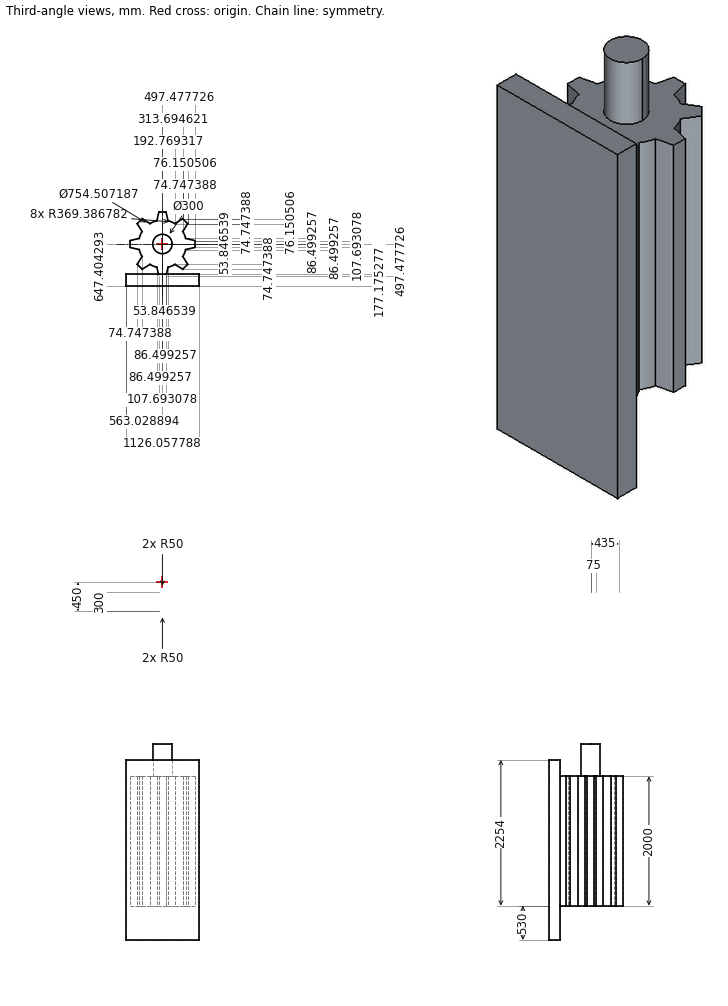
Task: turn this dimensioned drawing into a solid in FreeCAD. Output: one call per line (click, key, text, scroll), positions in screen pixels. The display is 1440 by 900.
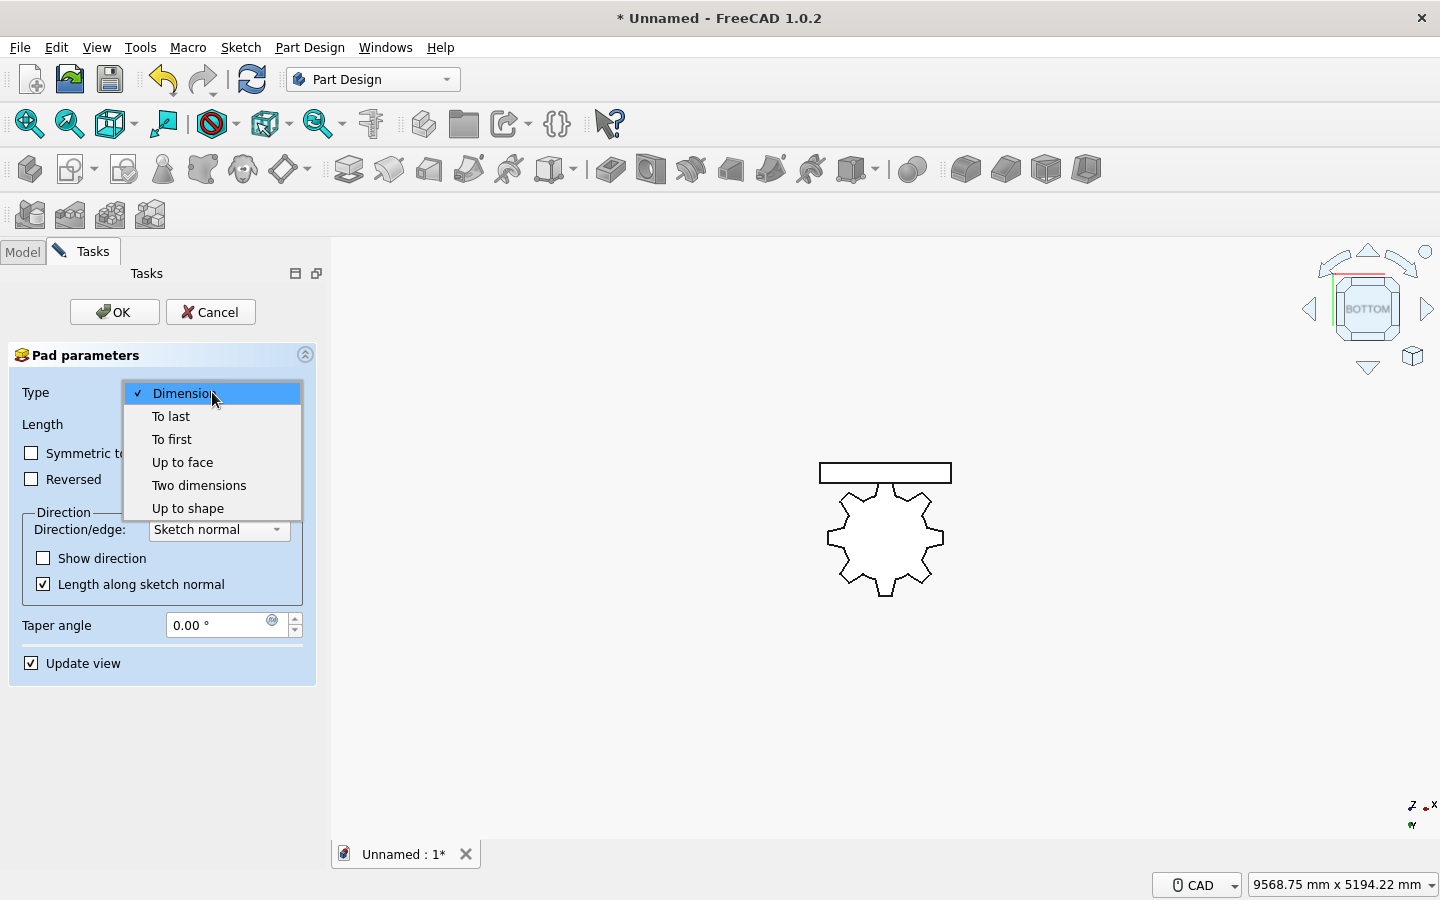
click(212, 486)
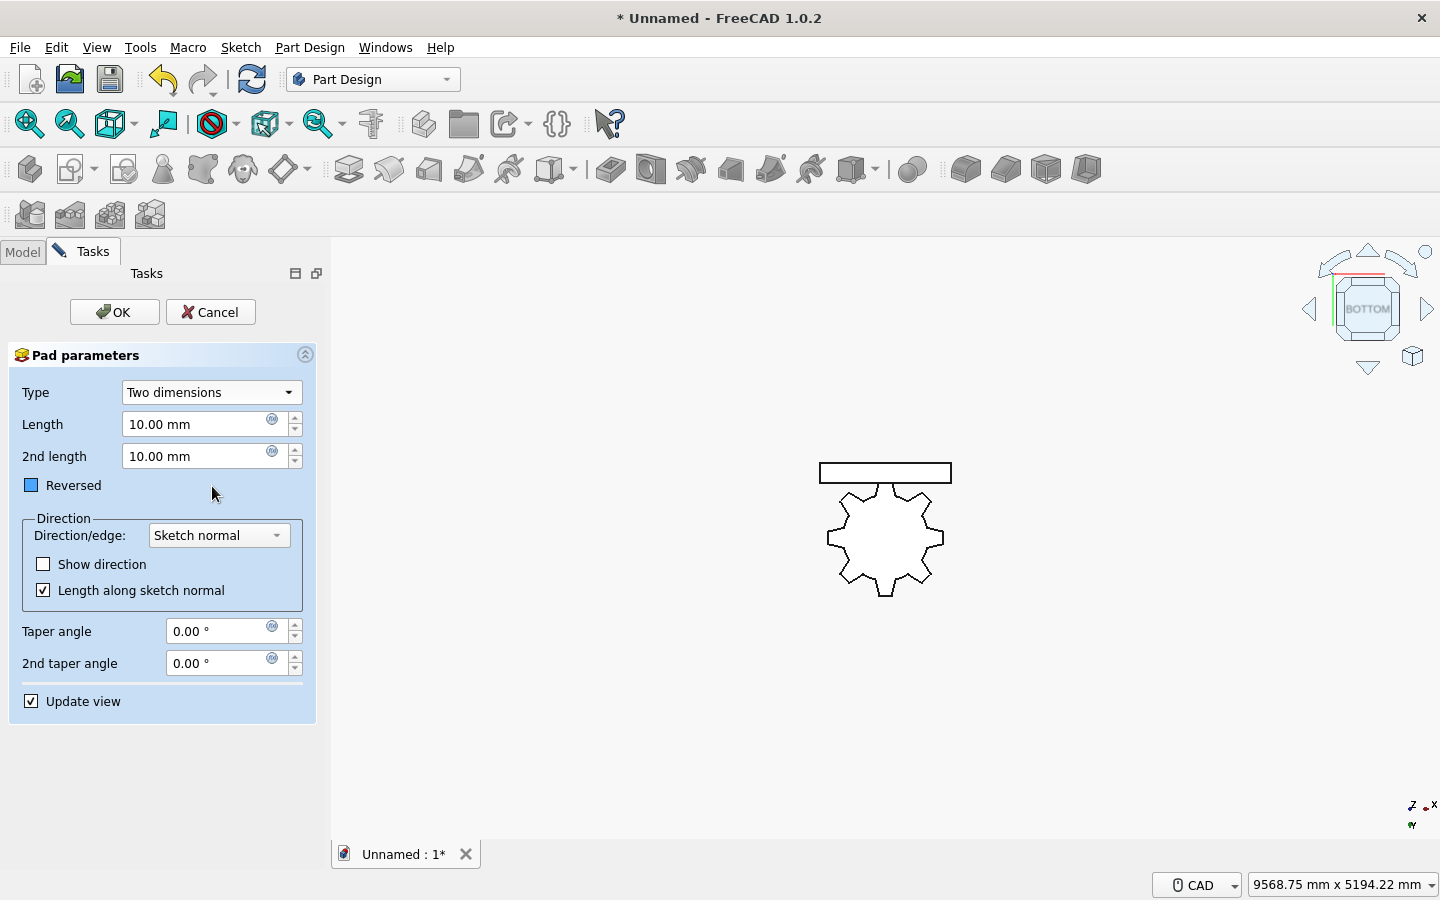
triple_click(204, 424)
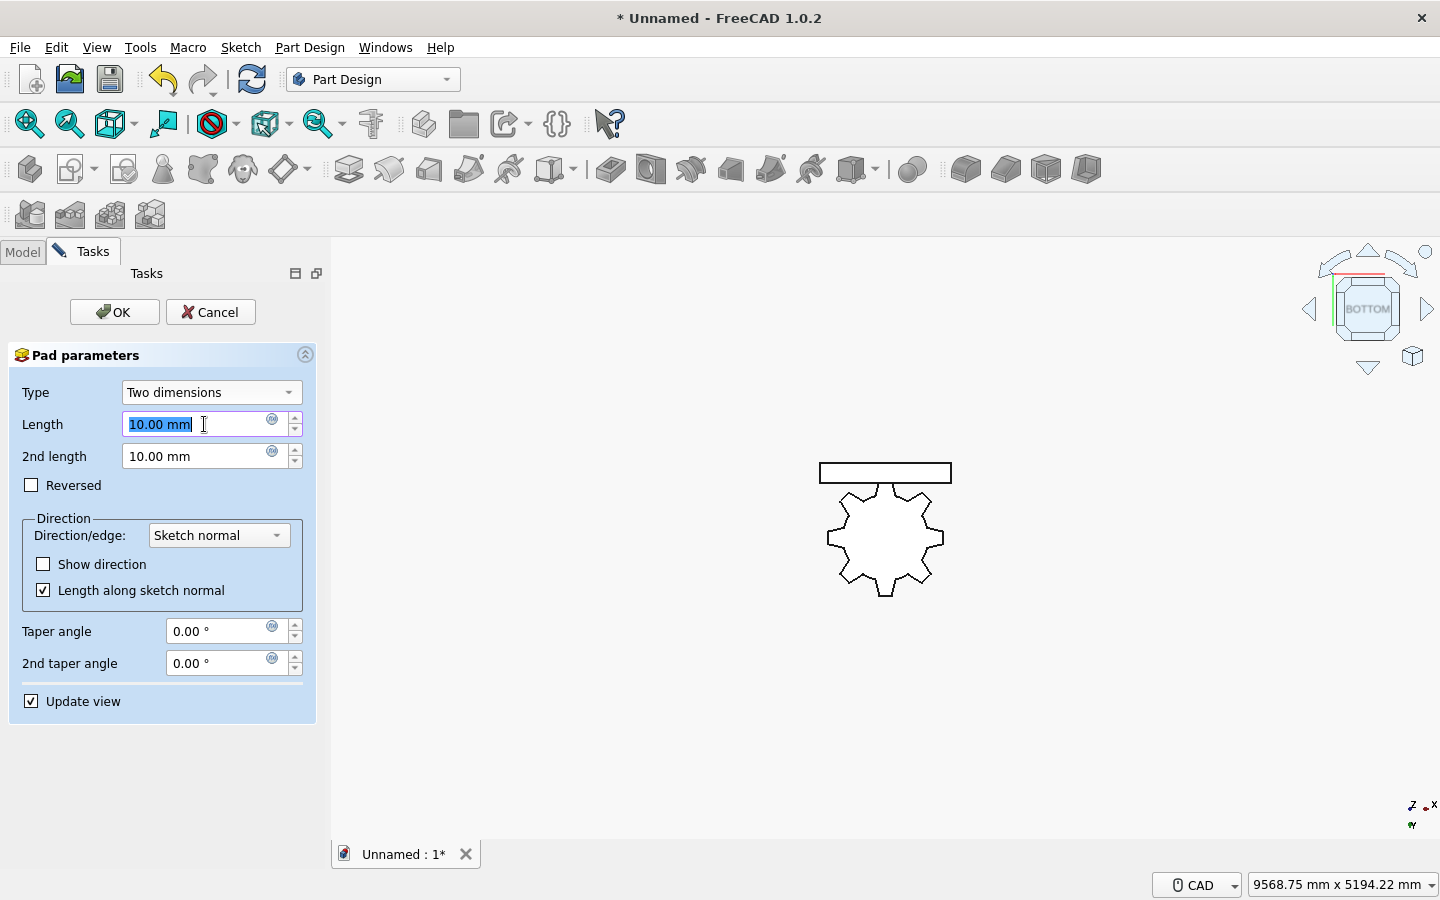
text(530)
key(Tab)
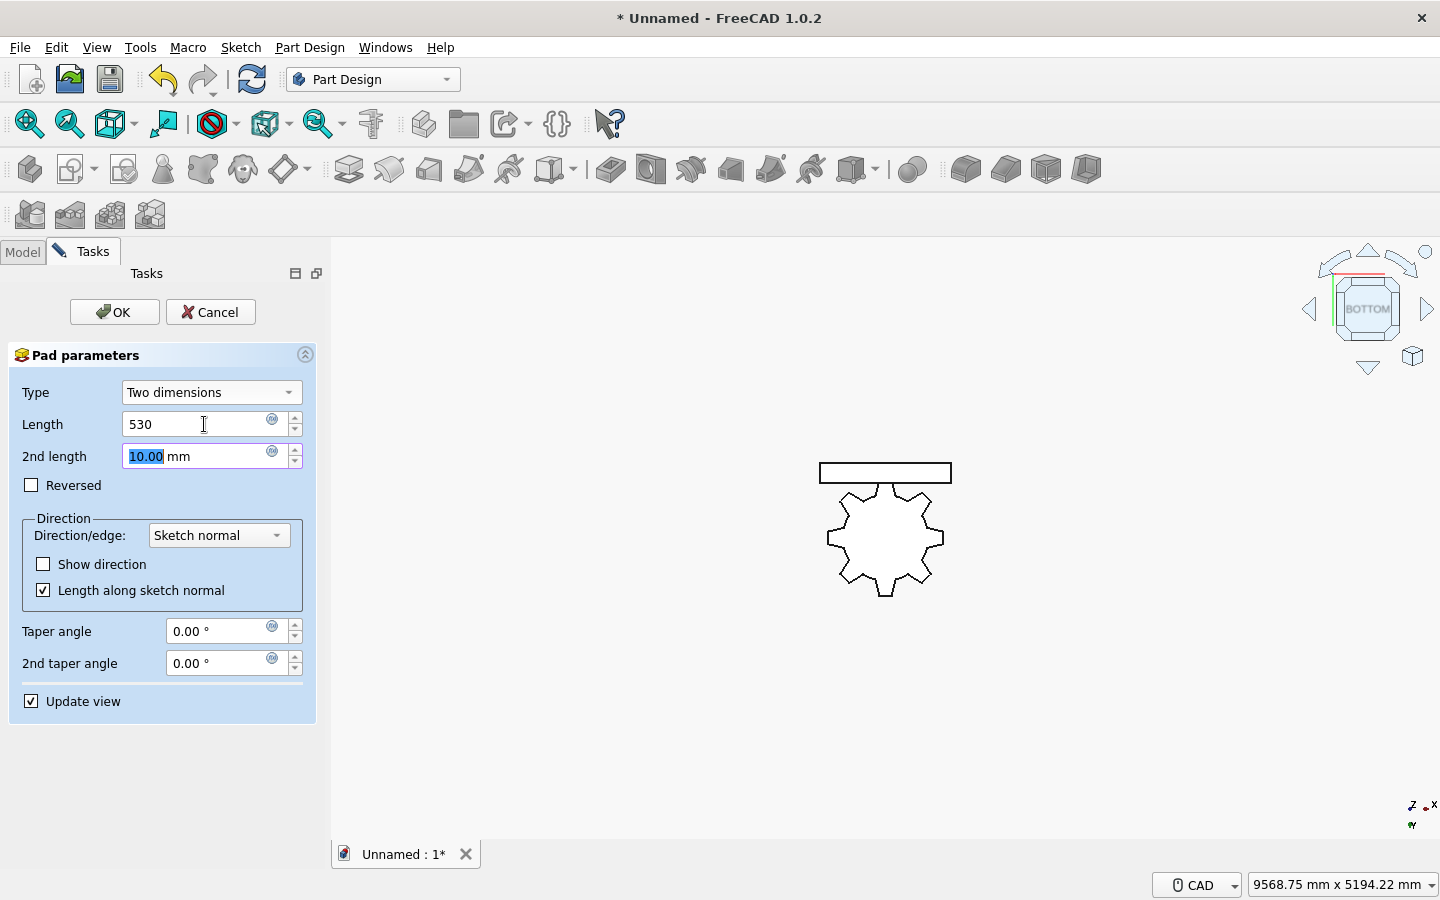
text(2254)
key(Tab)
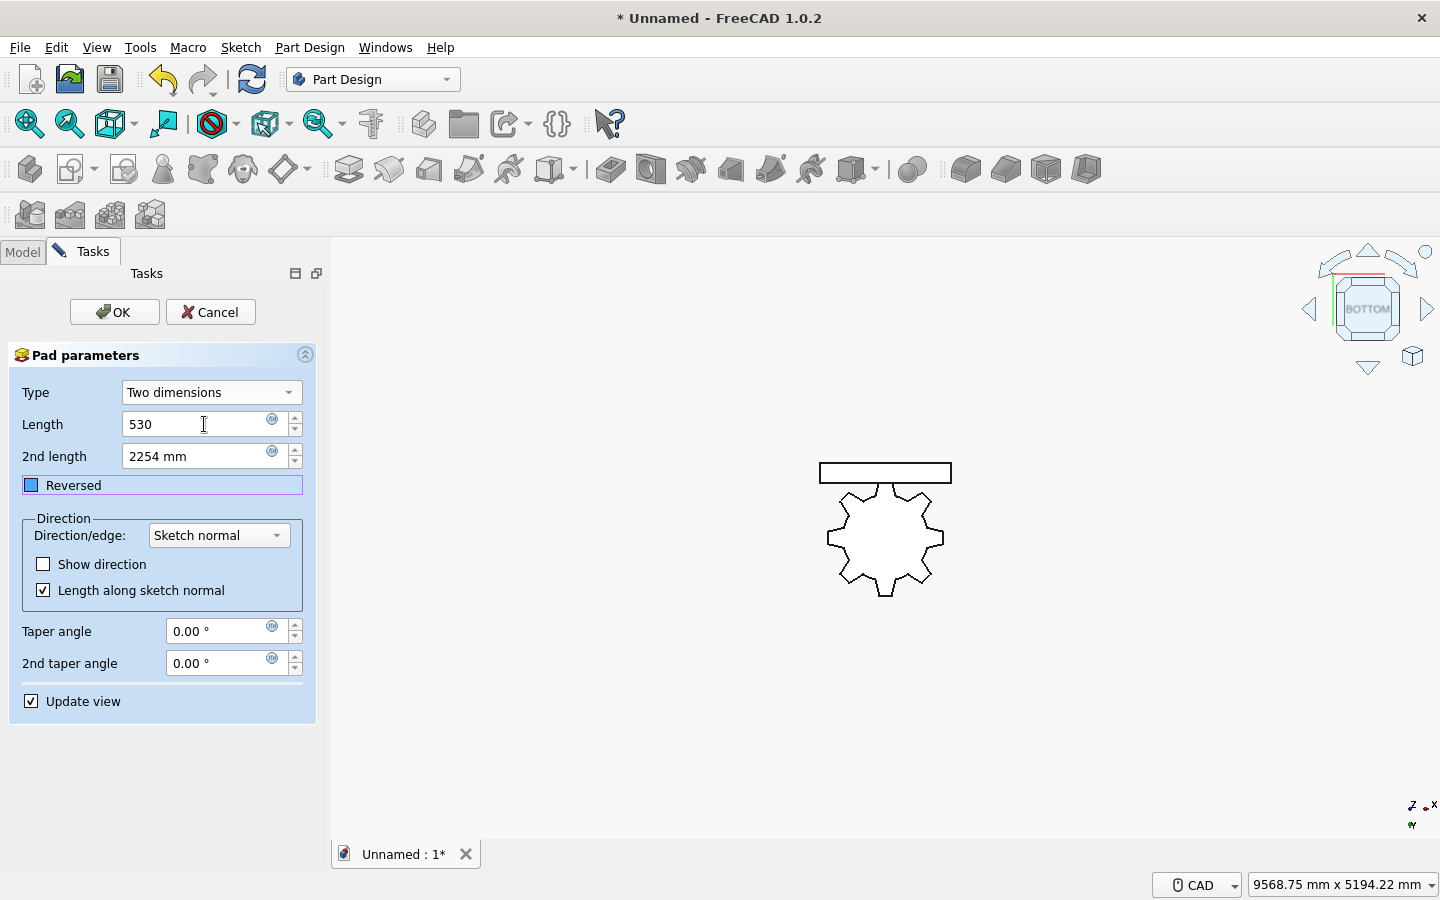
click(115, 312)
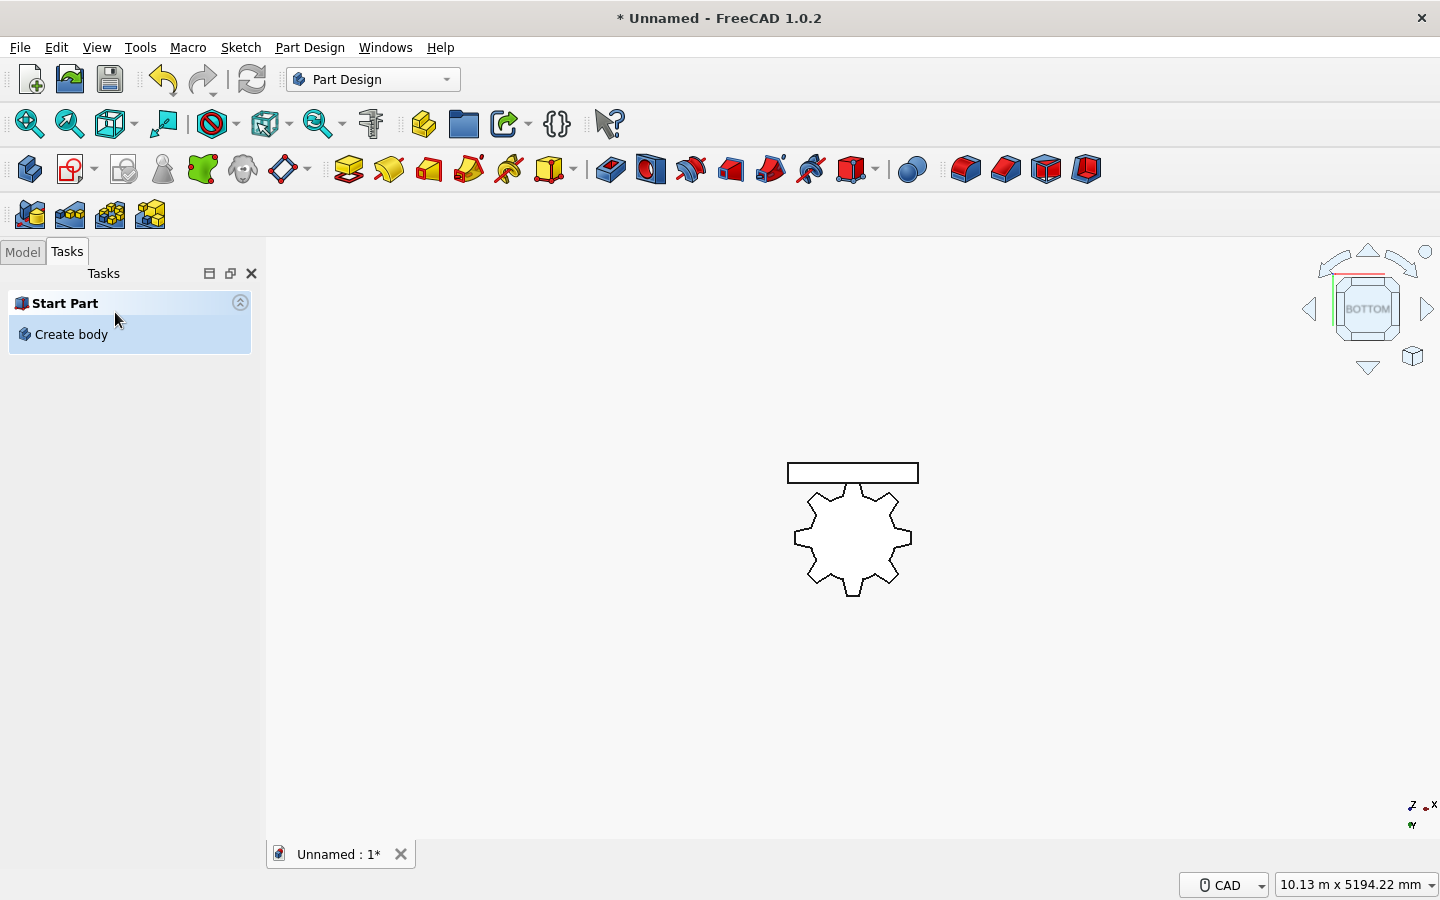
click(30, 124)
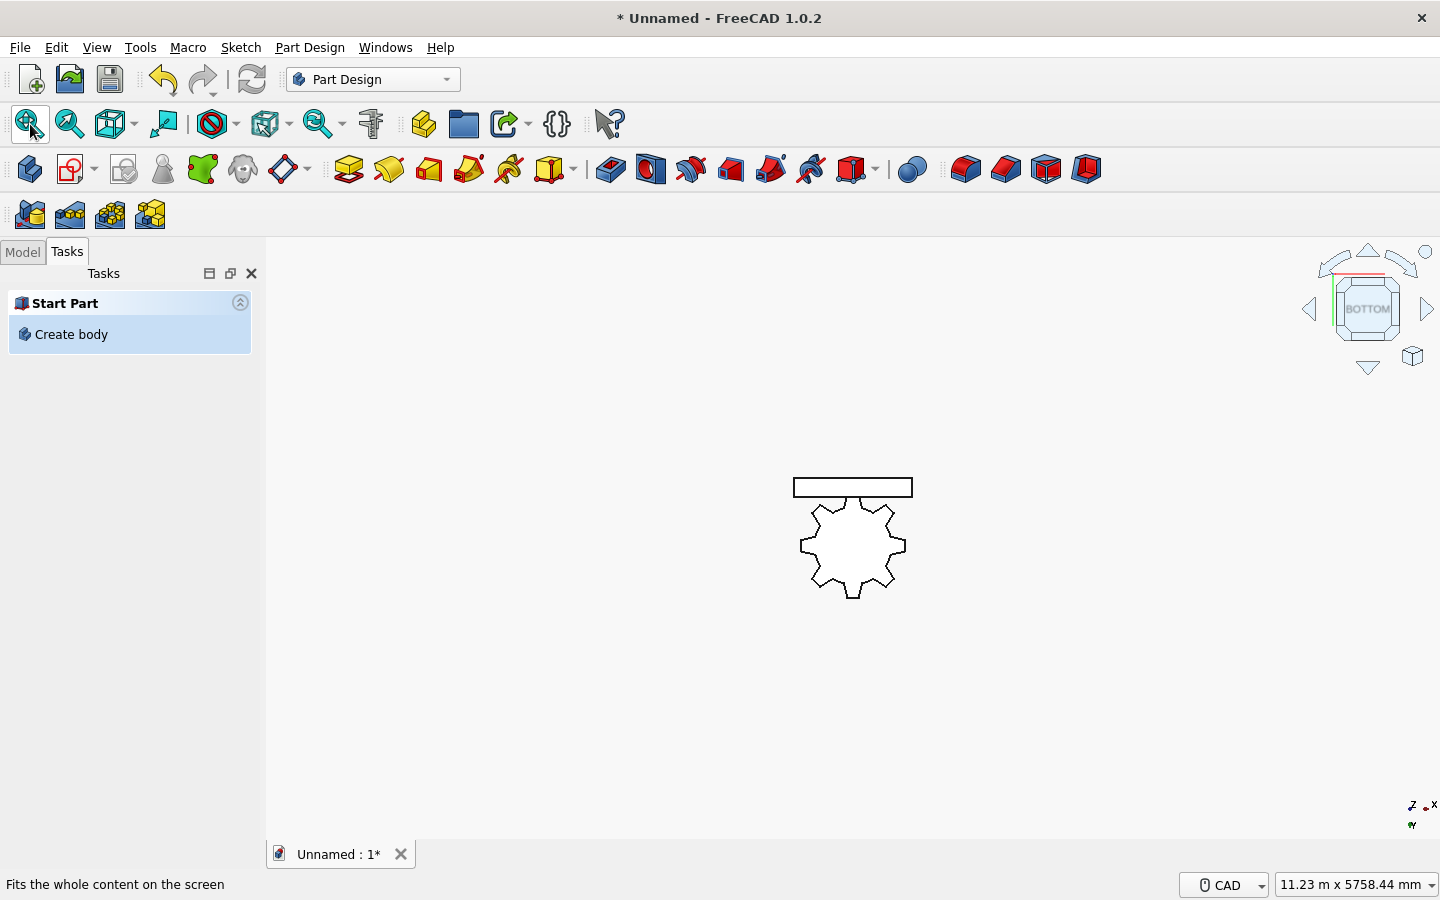
key(4)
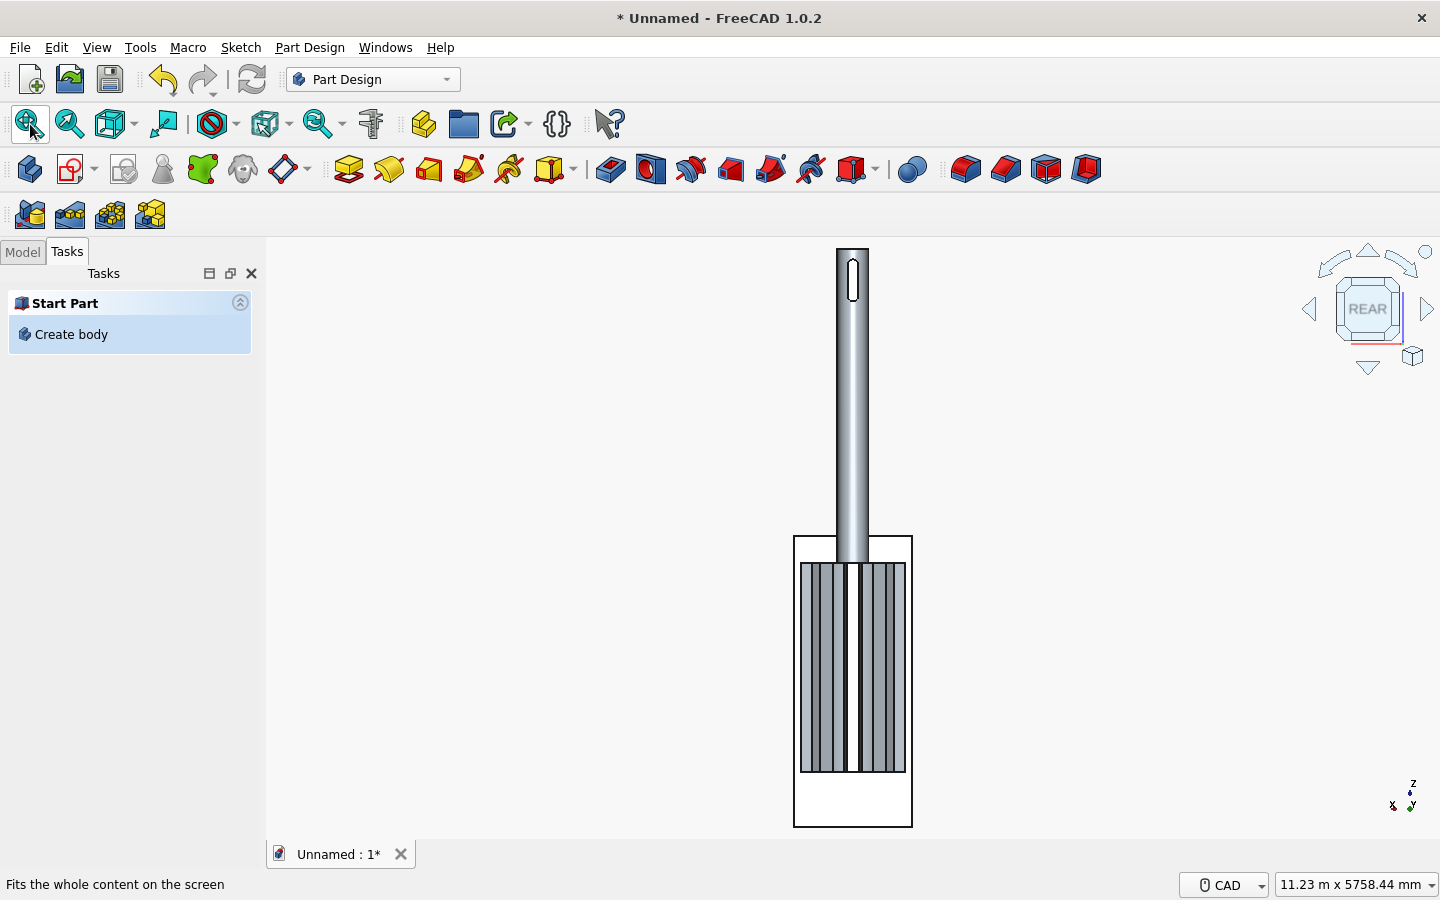
scroll(853, 291, up, 5)